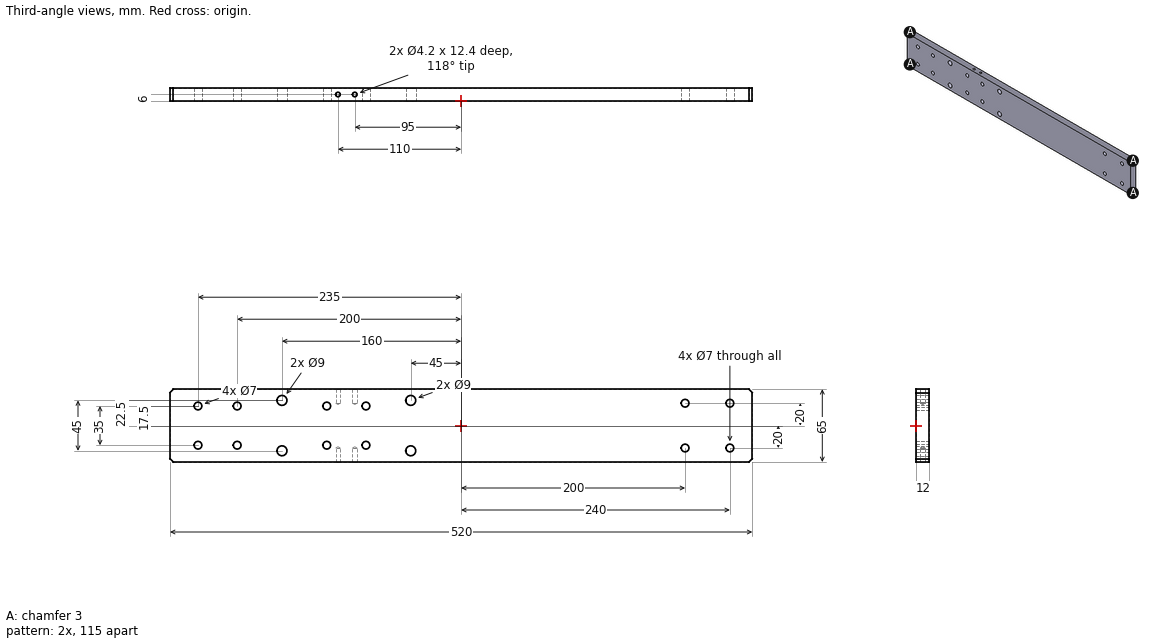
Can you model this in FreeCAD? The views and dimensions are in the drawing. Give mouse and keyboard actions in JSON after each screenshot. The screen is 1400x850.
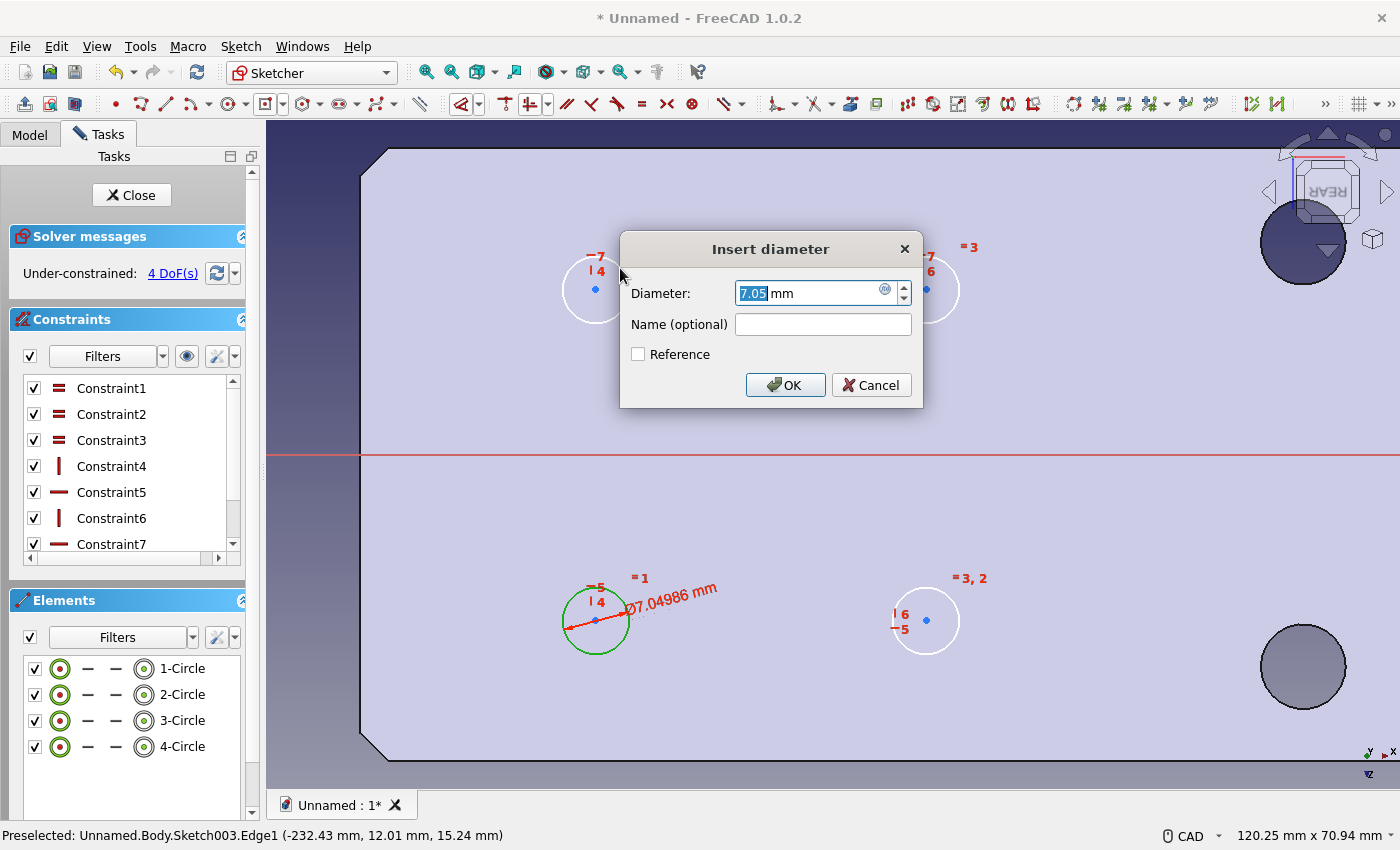
{"action": "type", "text": "7"}
{"action": "key", "text": "Return"}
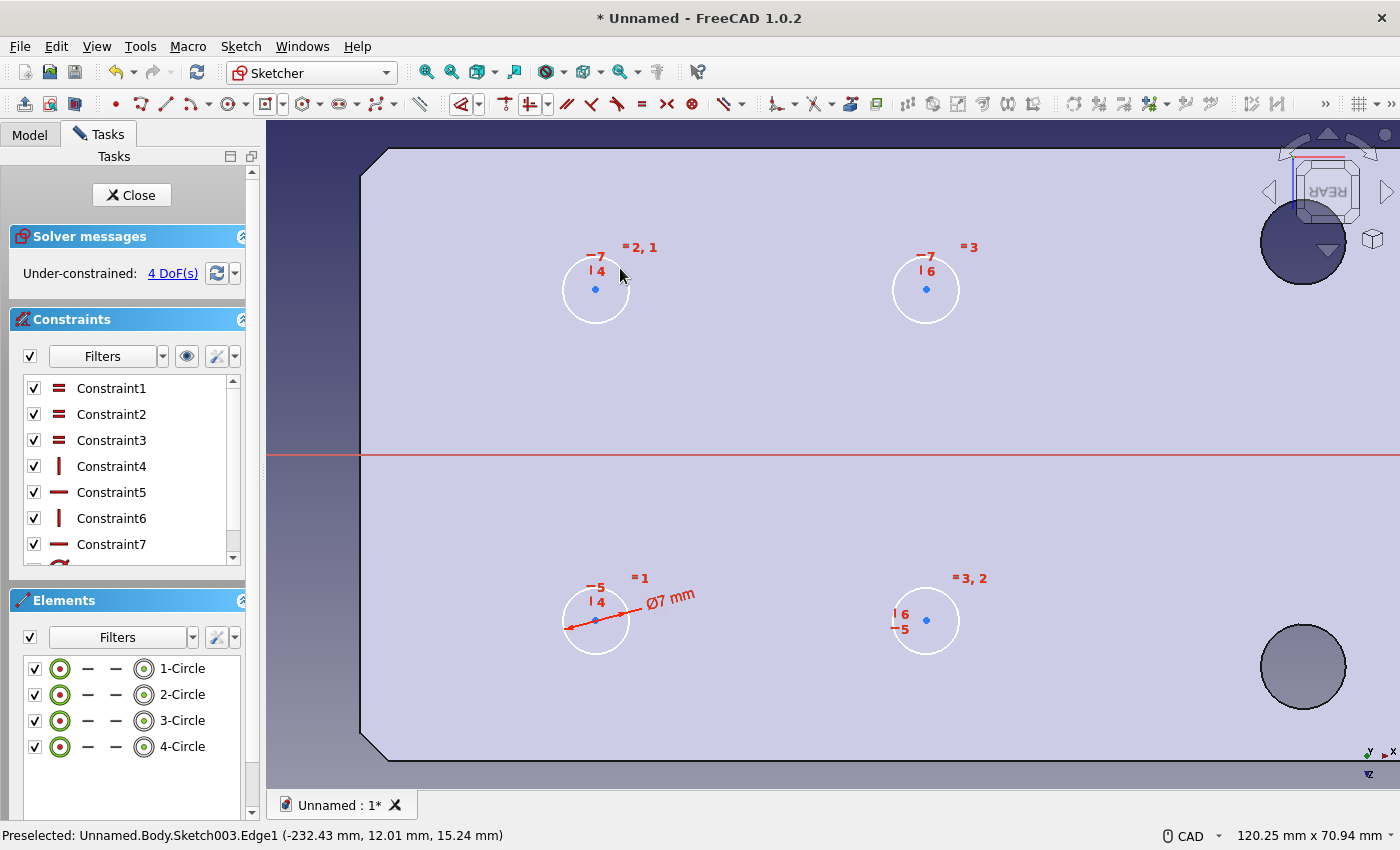
{"action": "left_click", "coordinate": [596, 621]}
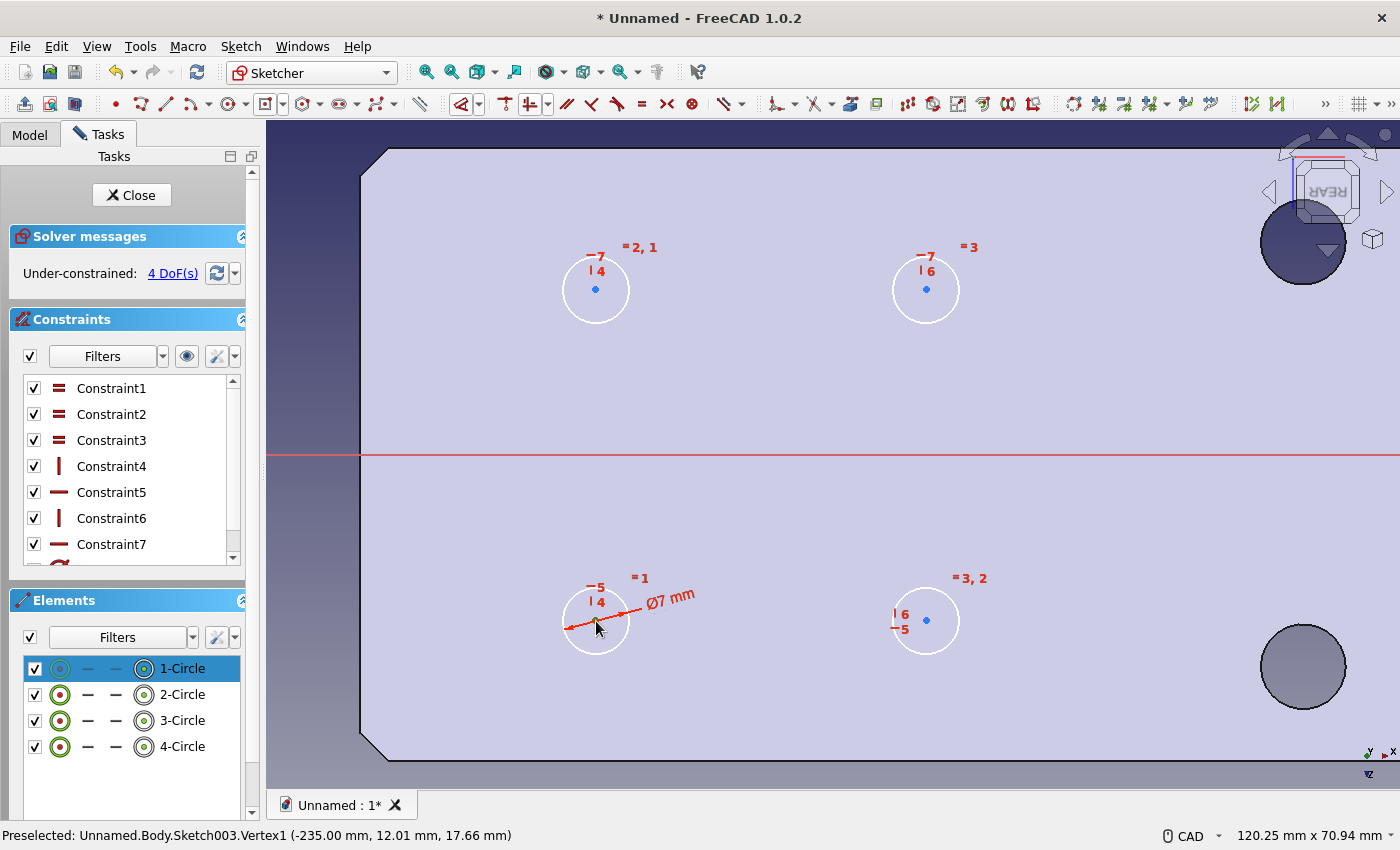
{"action": "left_click", "coordinate": [478, 104]}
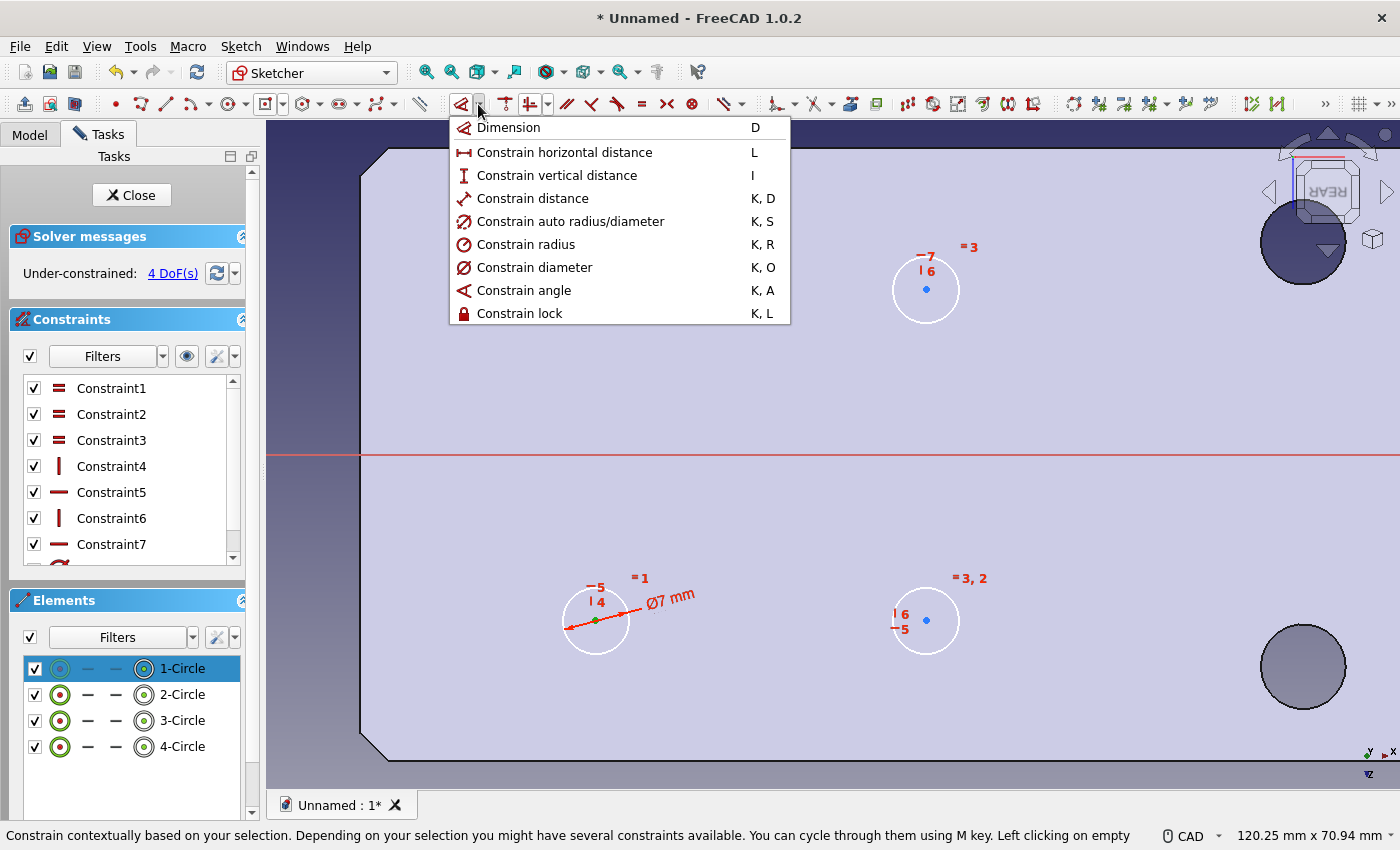
{"action": "left_click", "coordinate": [620, 152]}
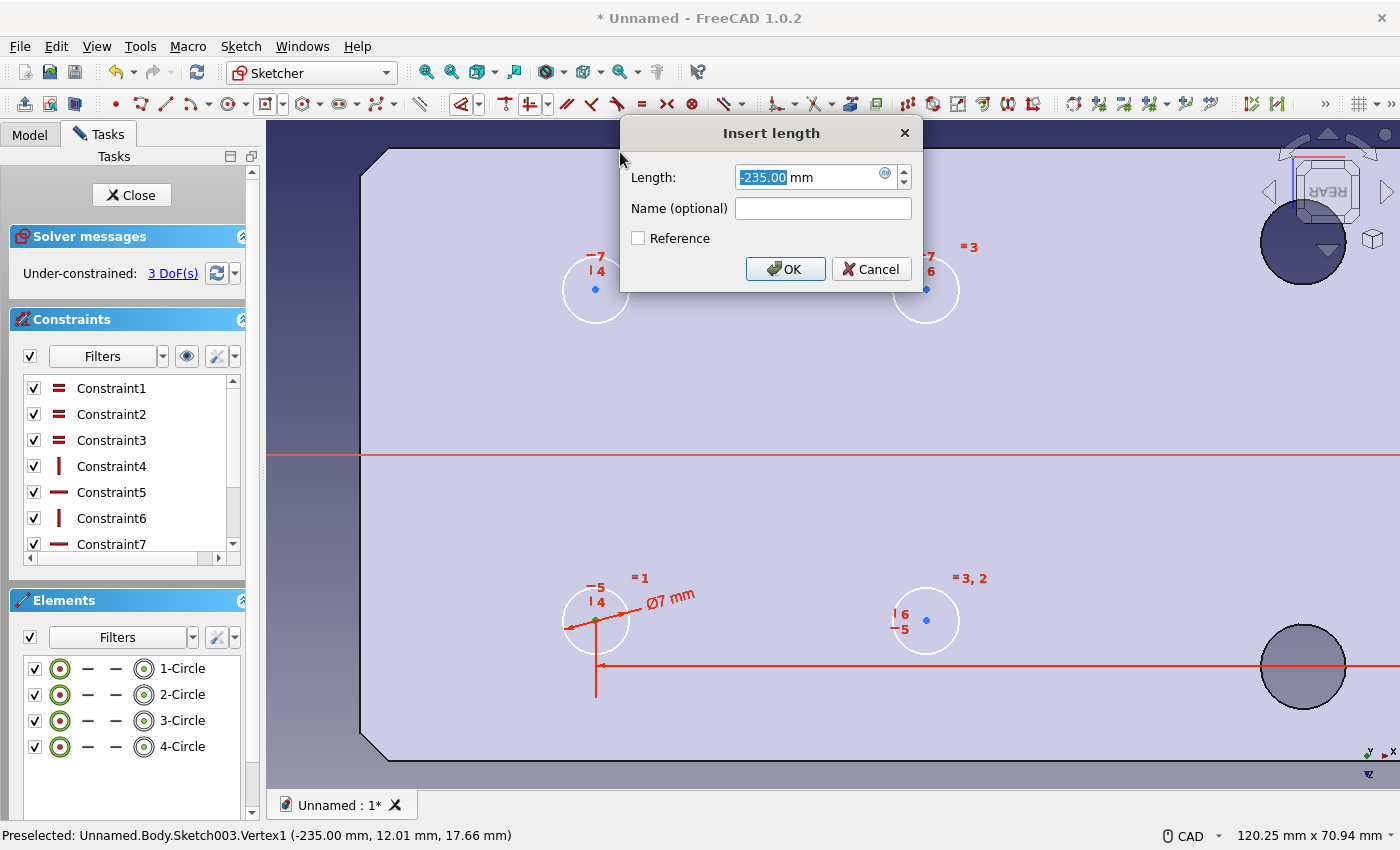
{"action": "type", "text": "-235"}
{"action": "key", "text": "Return"}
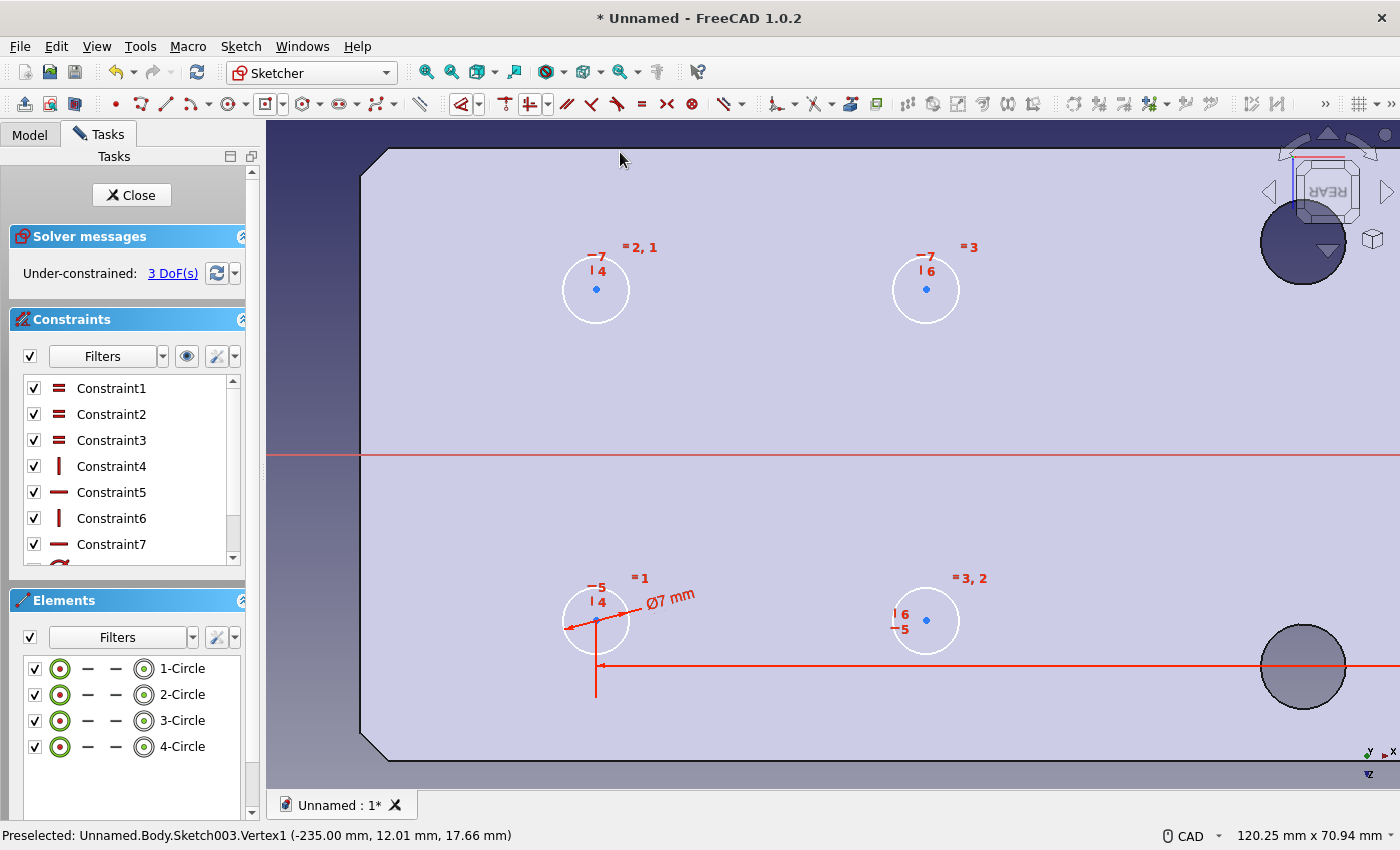
{"action": "left_click", "coordinate": [926, 621]}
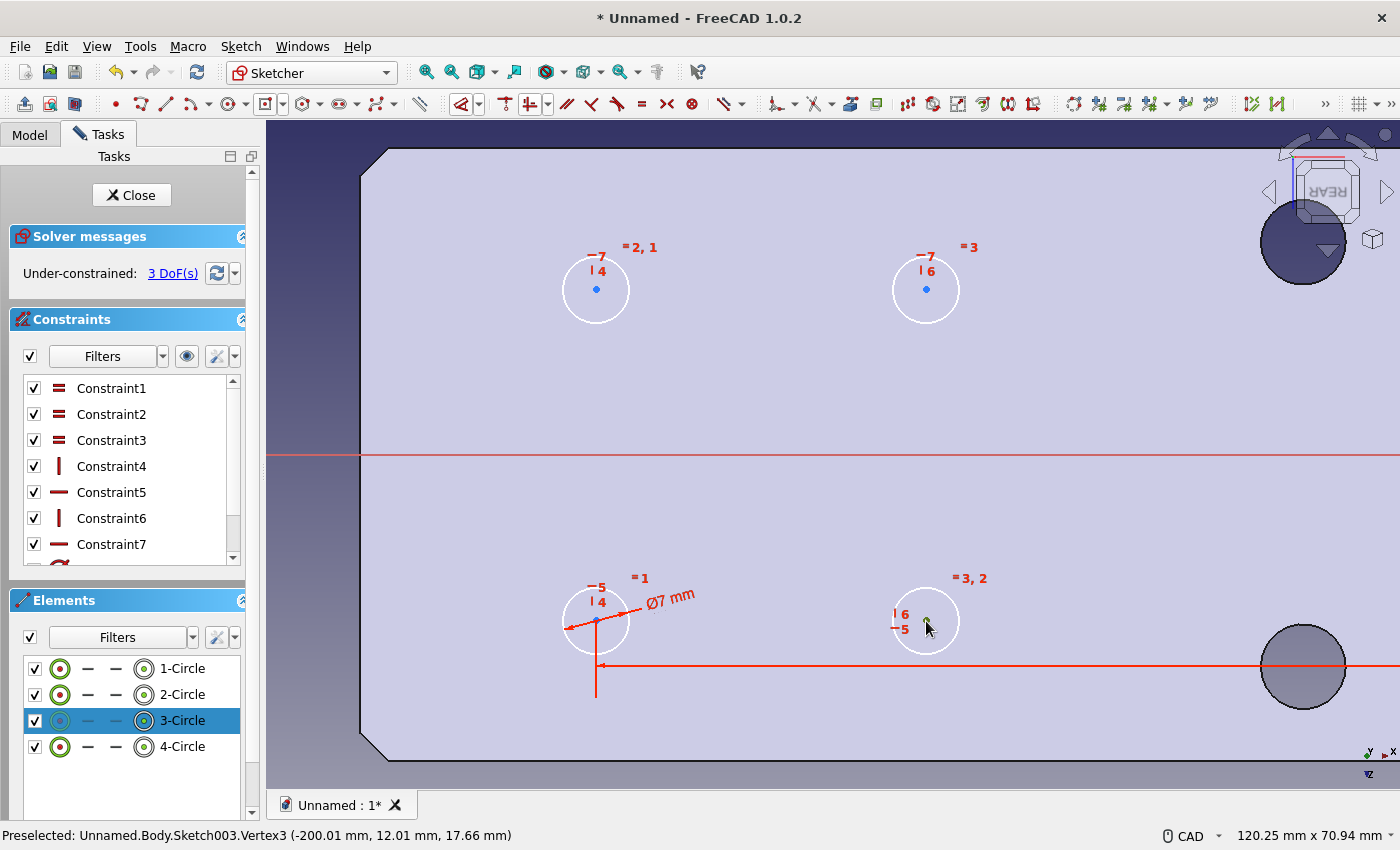
{"action": "left_click", "coordinate": [478, 104]}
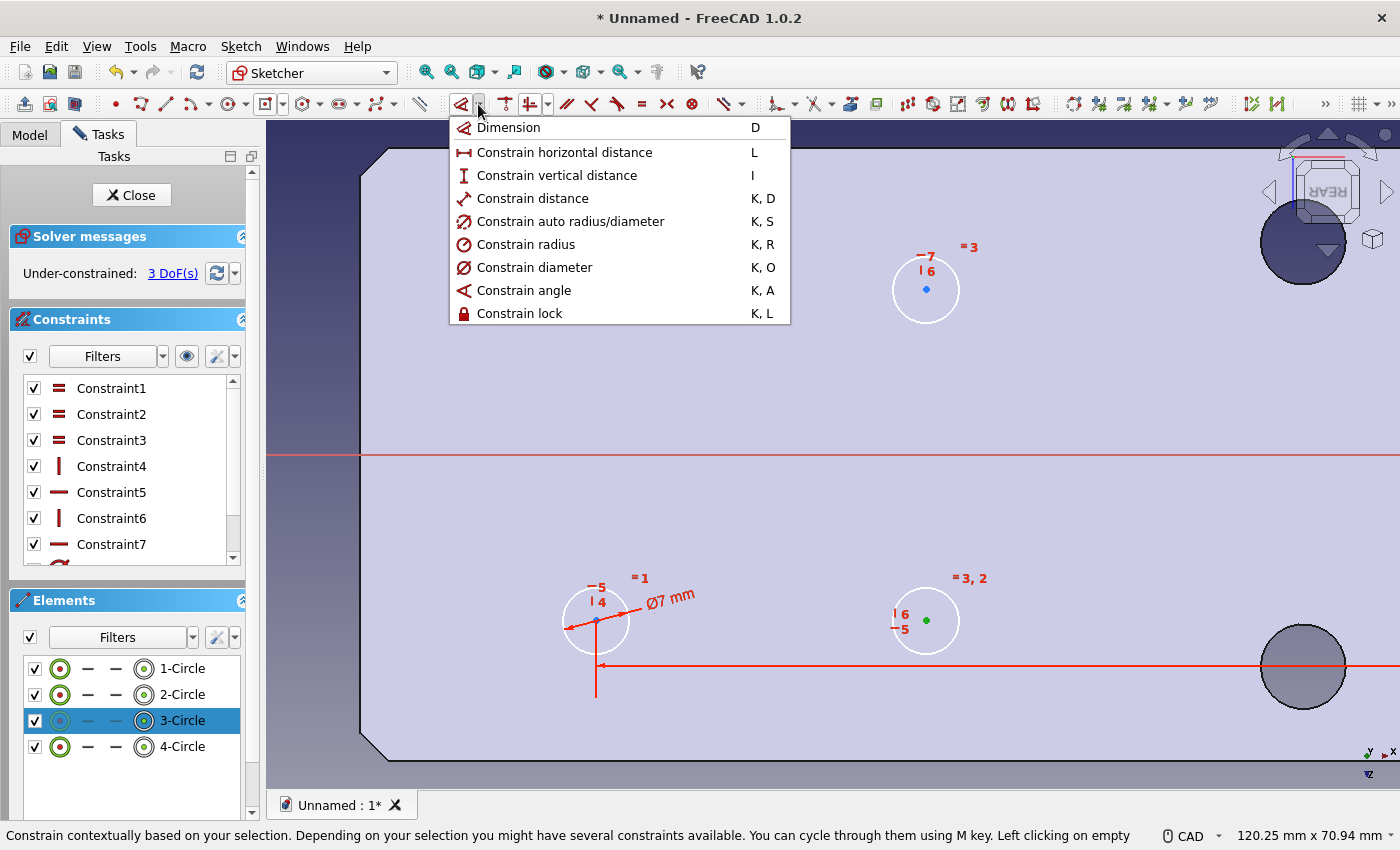
{"action": "left_click", "coordinate": [620, 152]}